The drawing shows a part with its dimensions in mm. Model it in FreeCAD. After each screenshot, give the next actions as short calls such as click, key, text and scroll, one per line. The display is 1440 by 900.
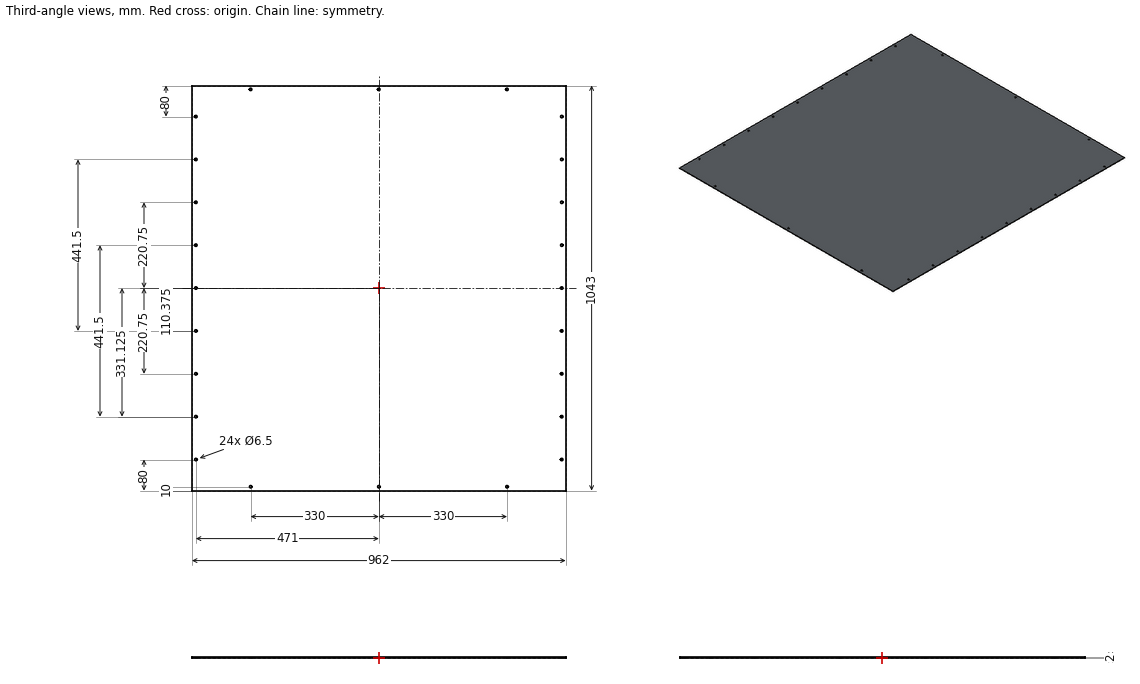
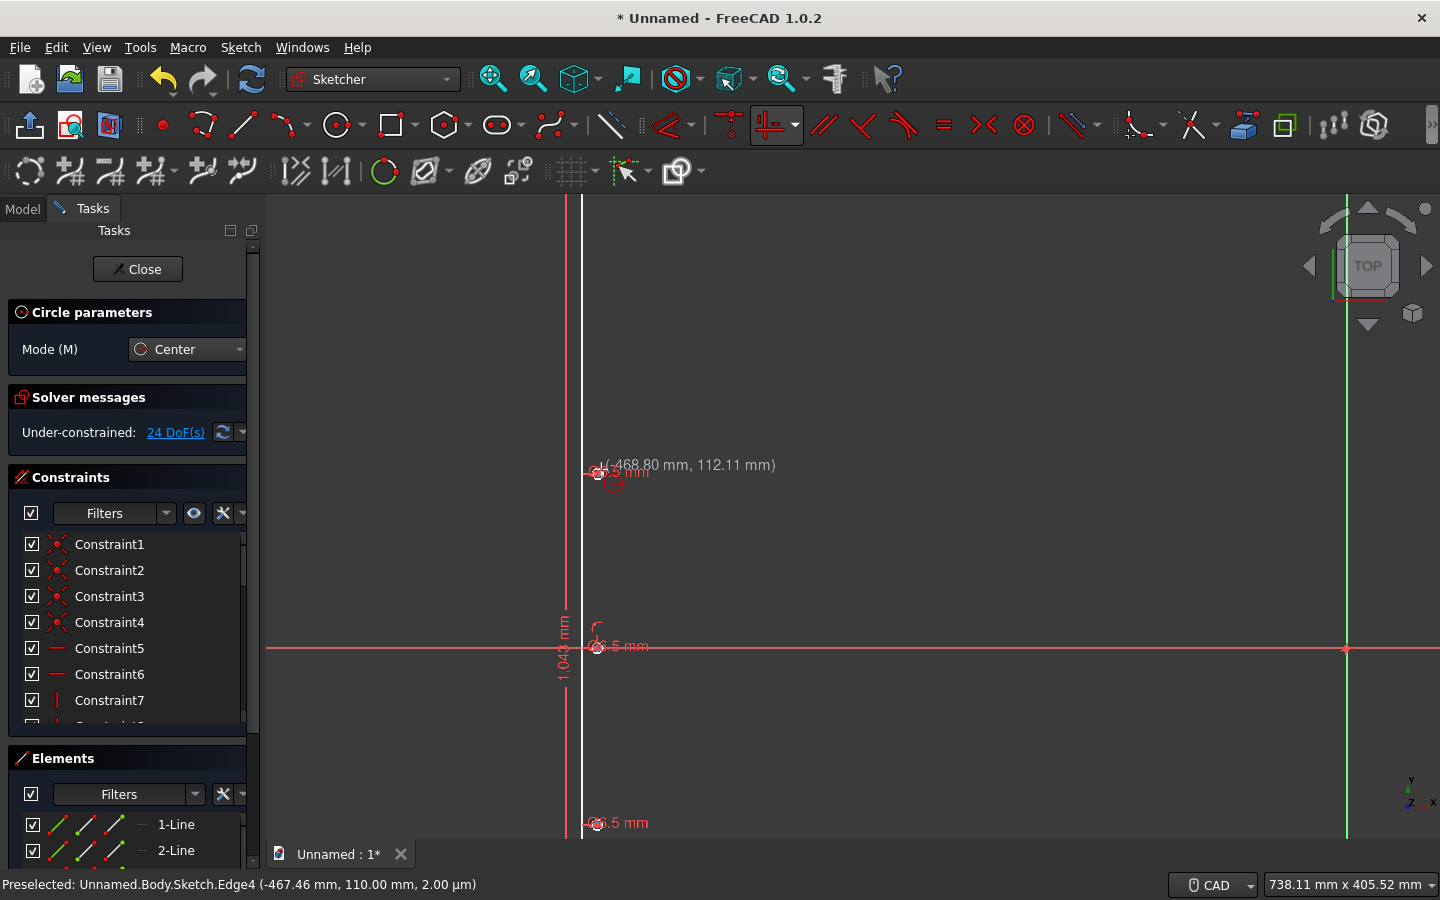
scroll(598, 297, up, 8)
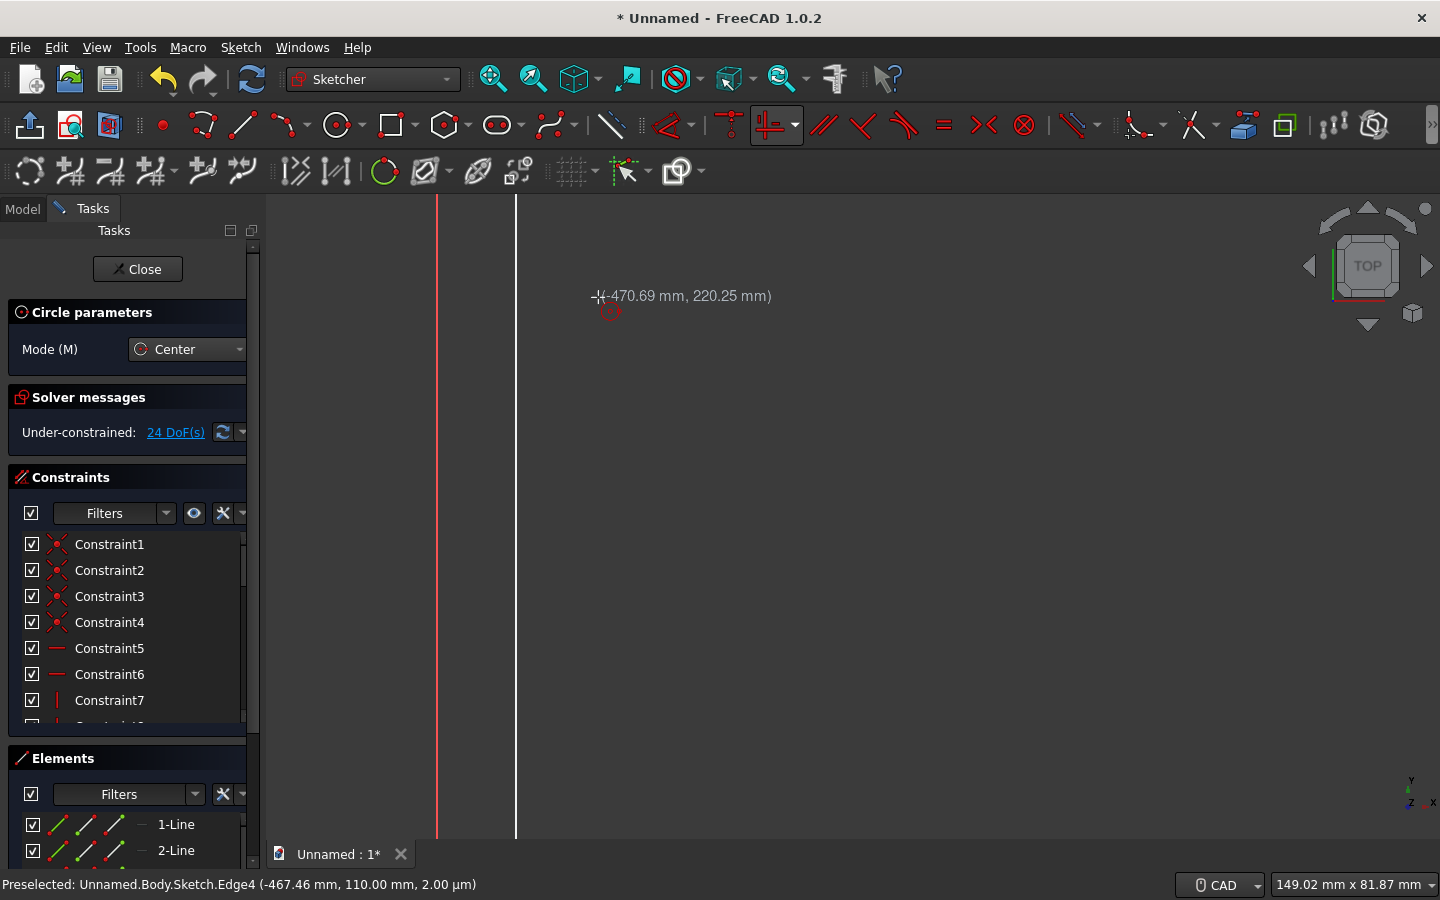
scroll(600, 437, down, 15)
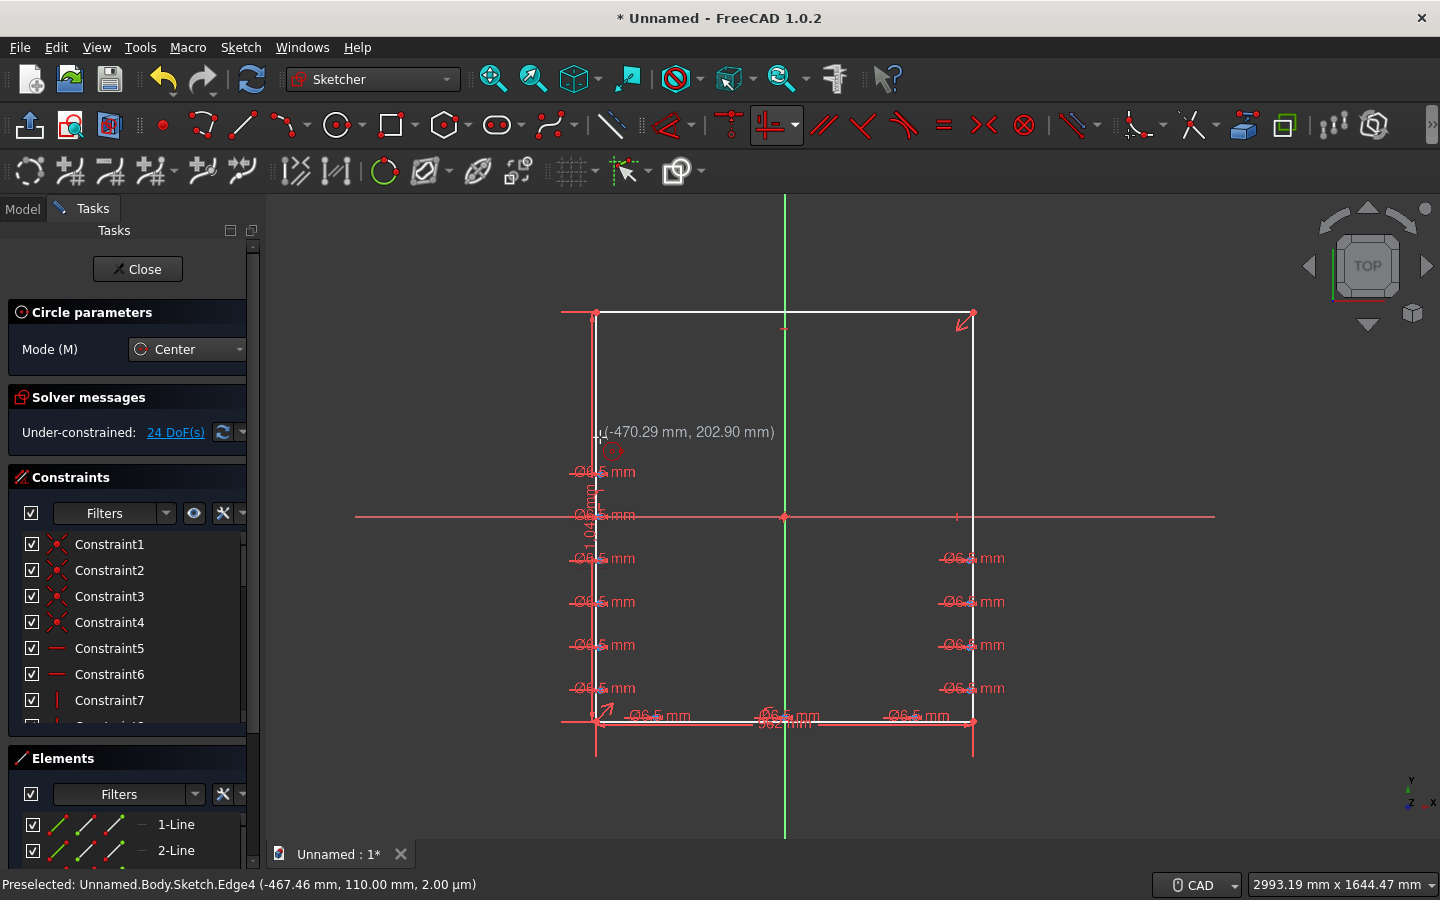
scroll(600, 430, up, 7)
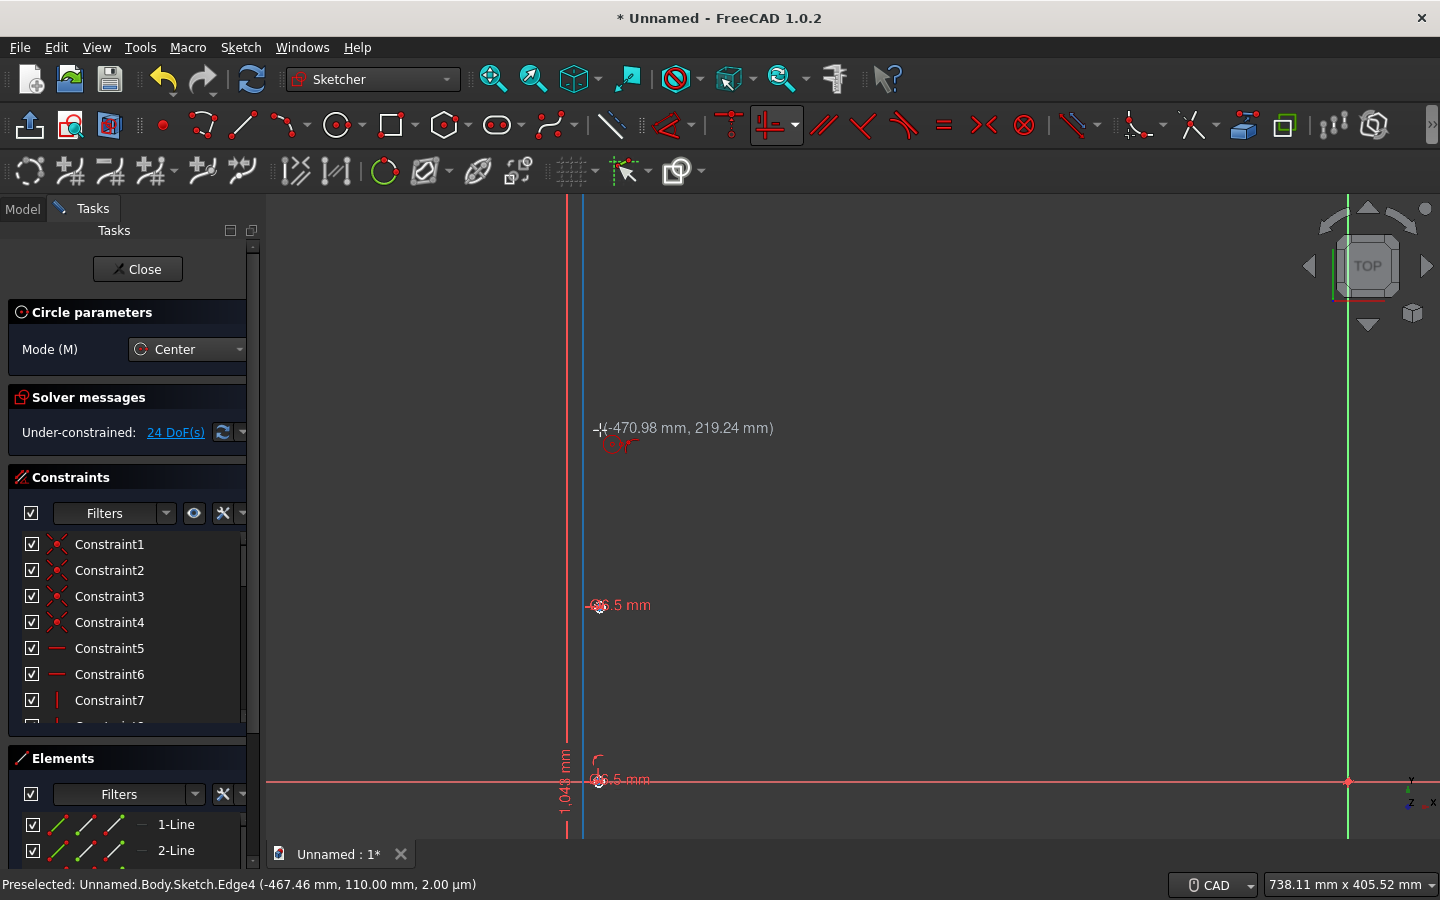
click(599, 431)
move(603, 427)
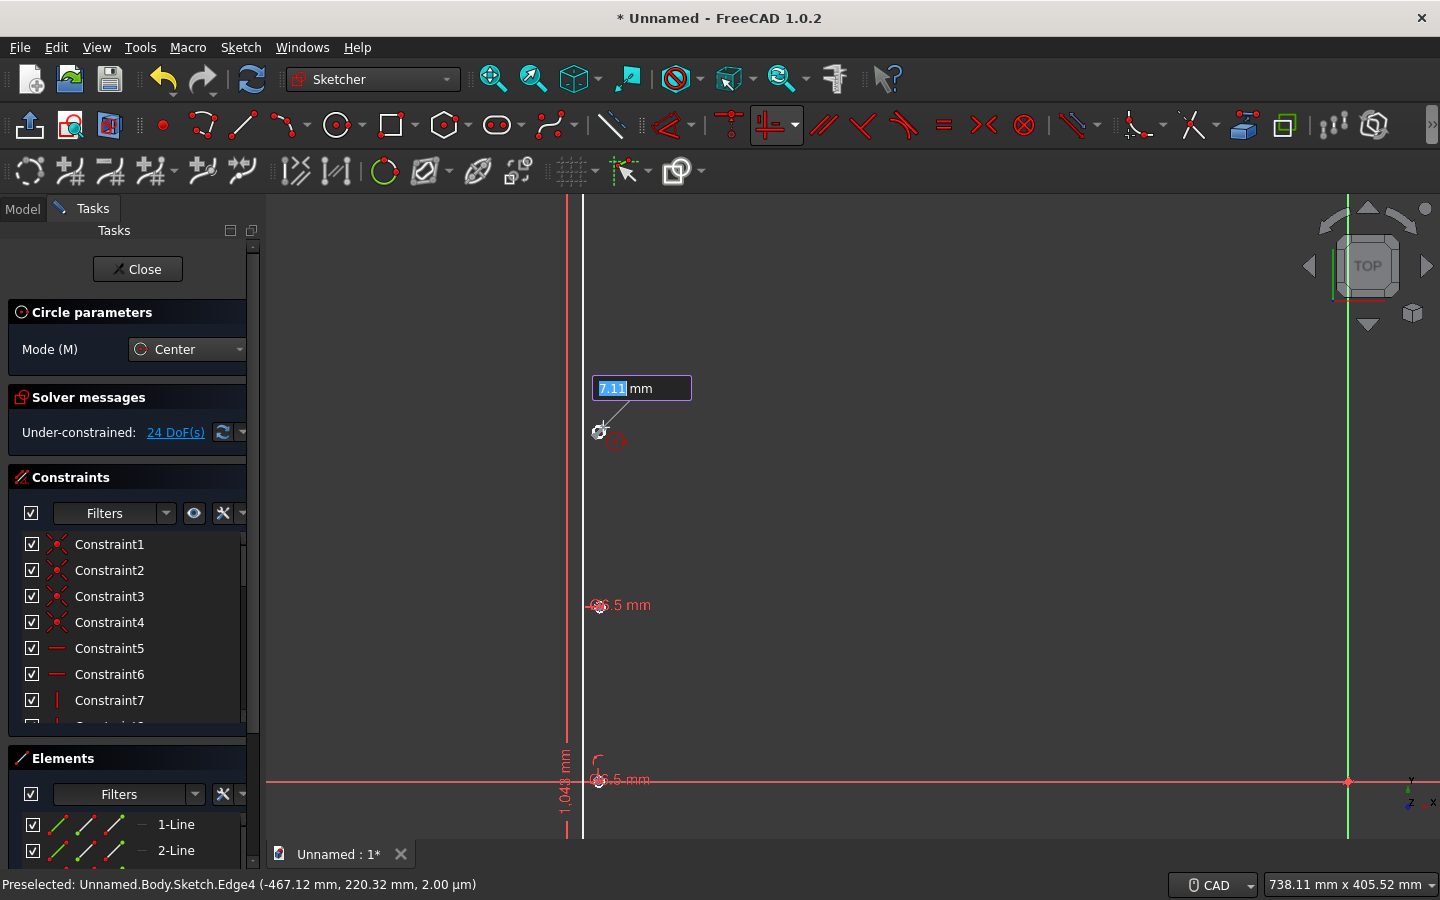
text(6.5)
key(Return)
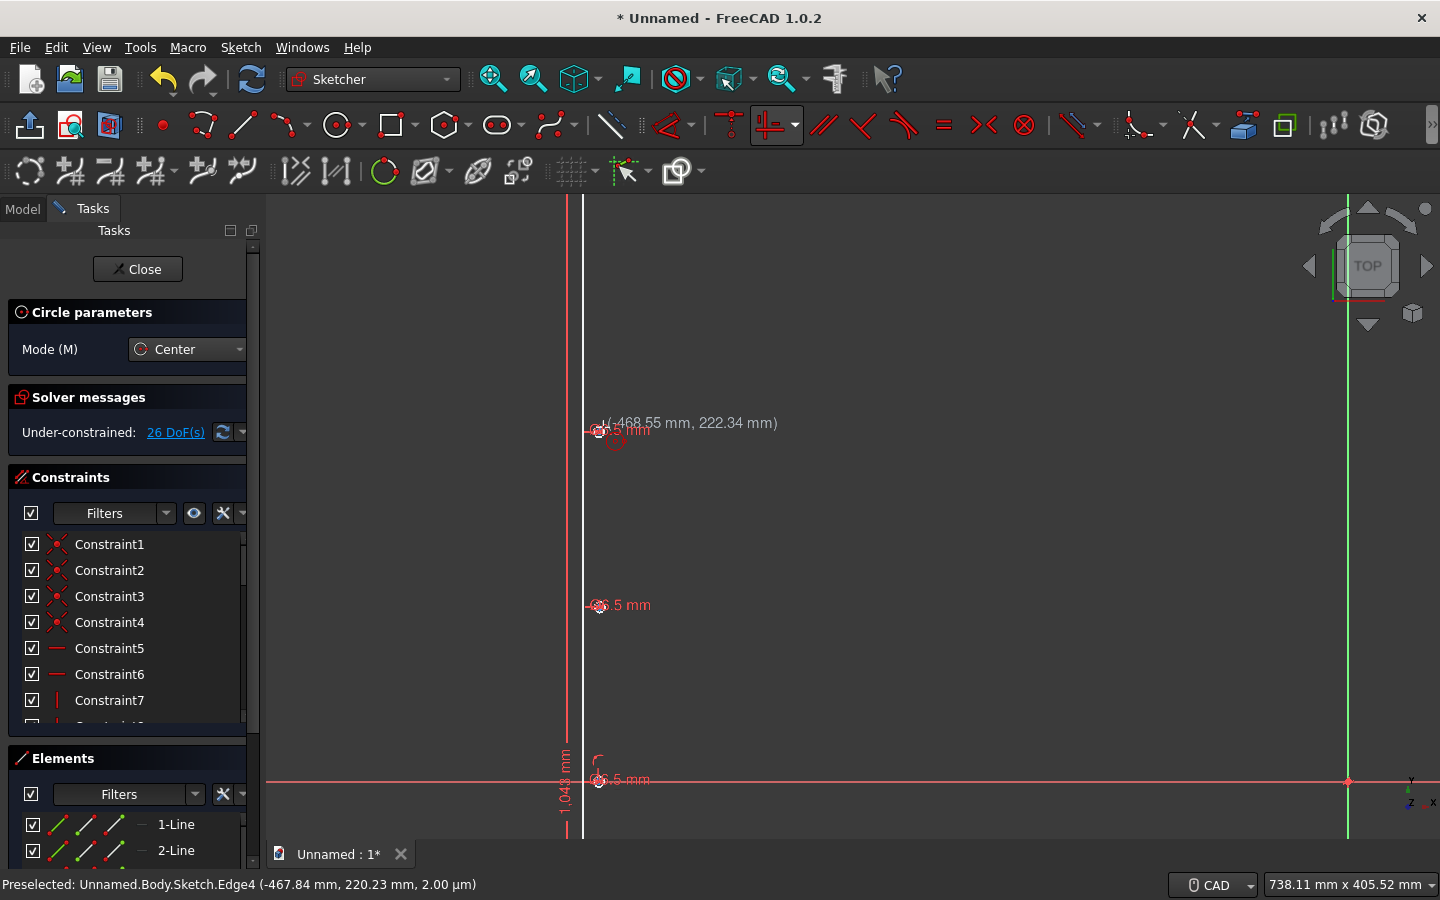
scroll(599, 255, up, 8)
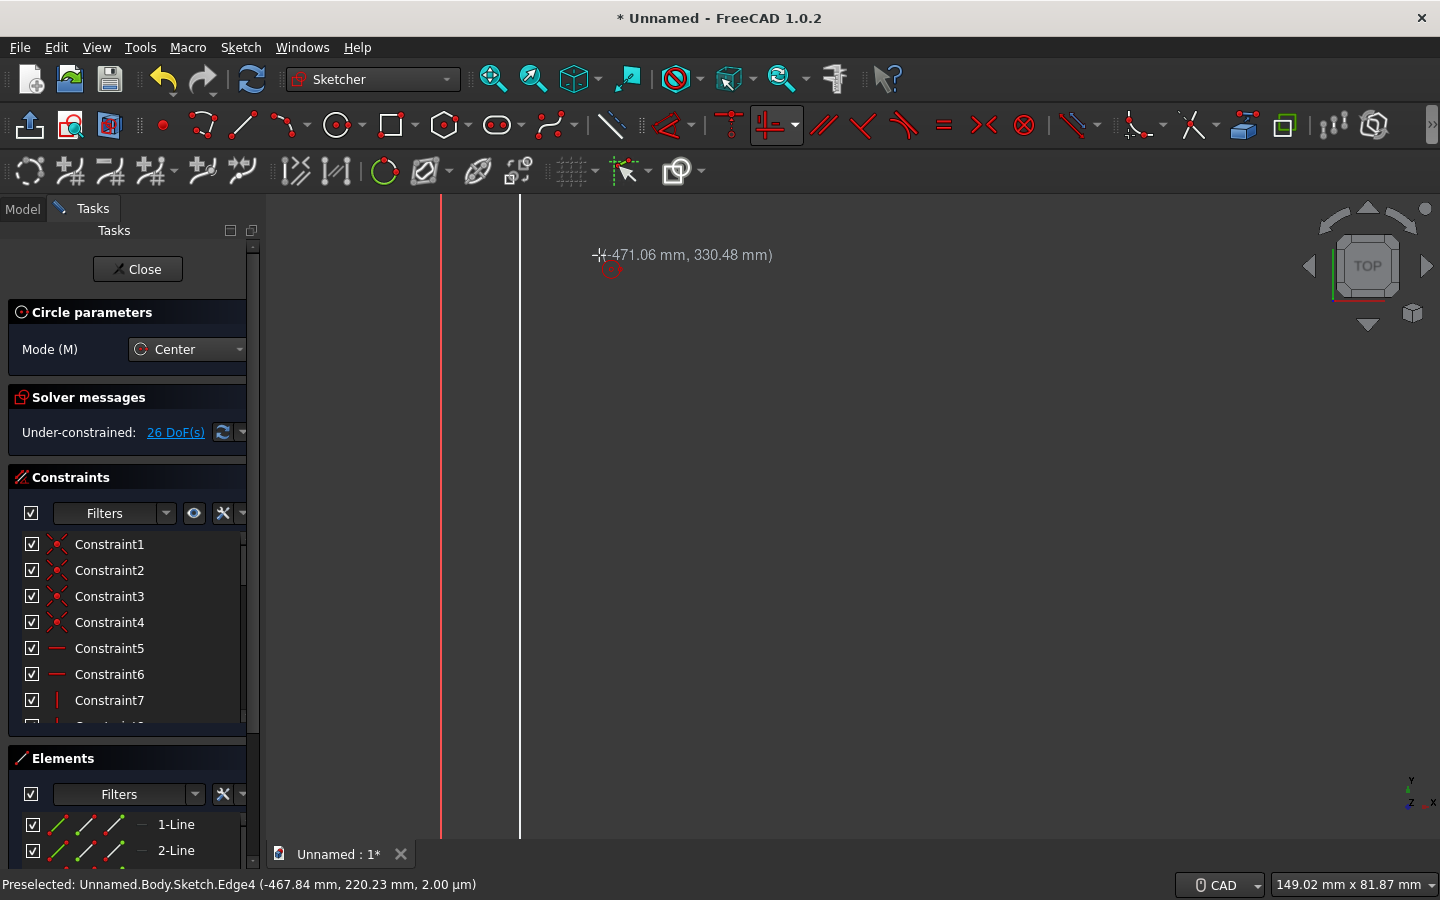
scroll(600, 394, down, 15)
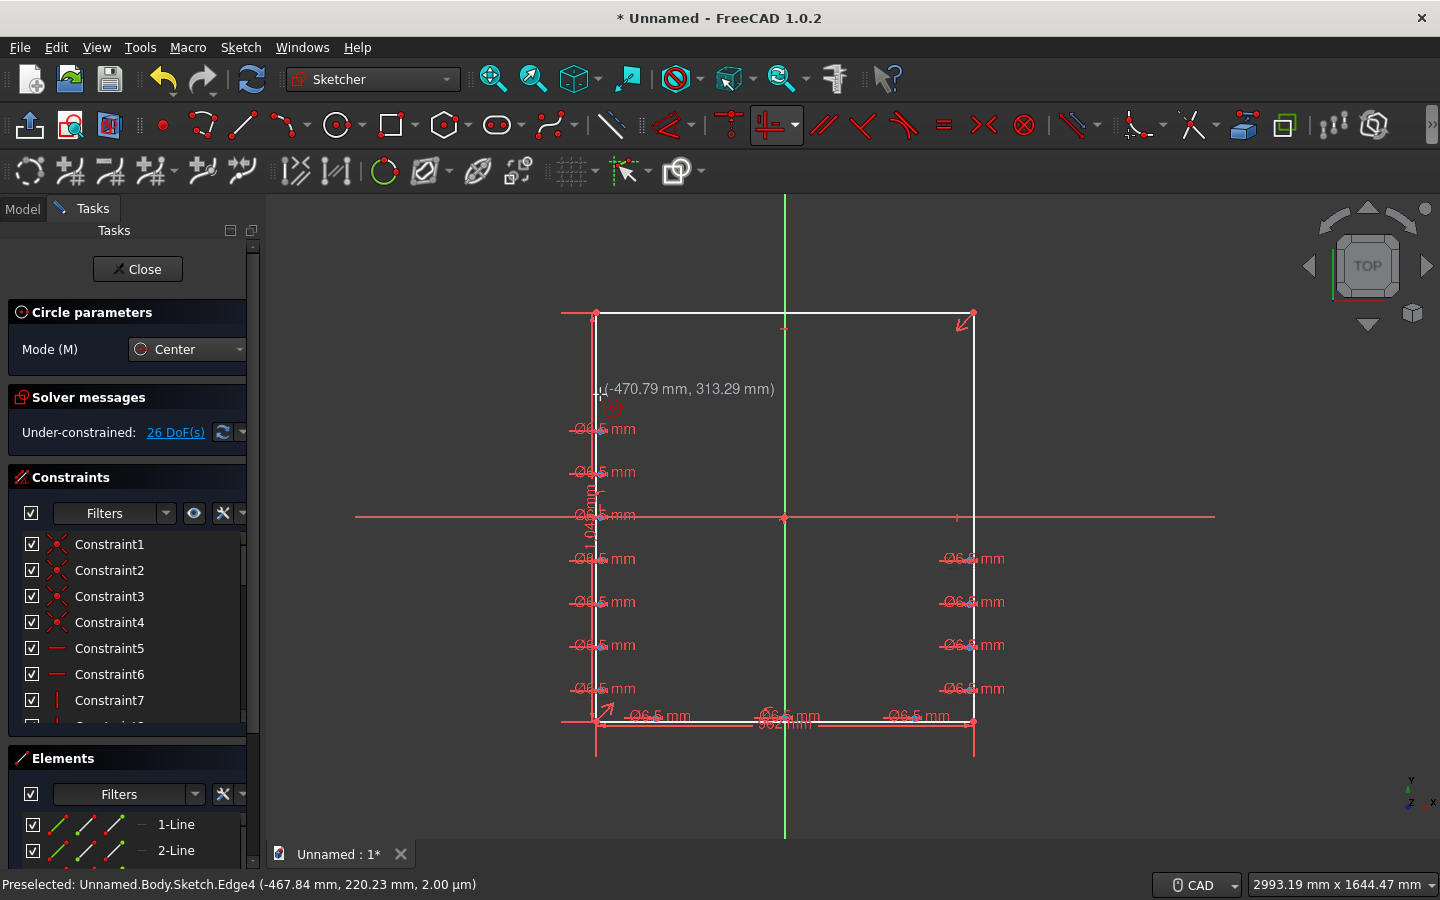
scroll(600, 387, up, 7)